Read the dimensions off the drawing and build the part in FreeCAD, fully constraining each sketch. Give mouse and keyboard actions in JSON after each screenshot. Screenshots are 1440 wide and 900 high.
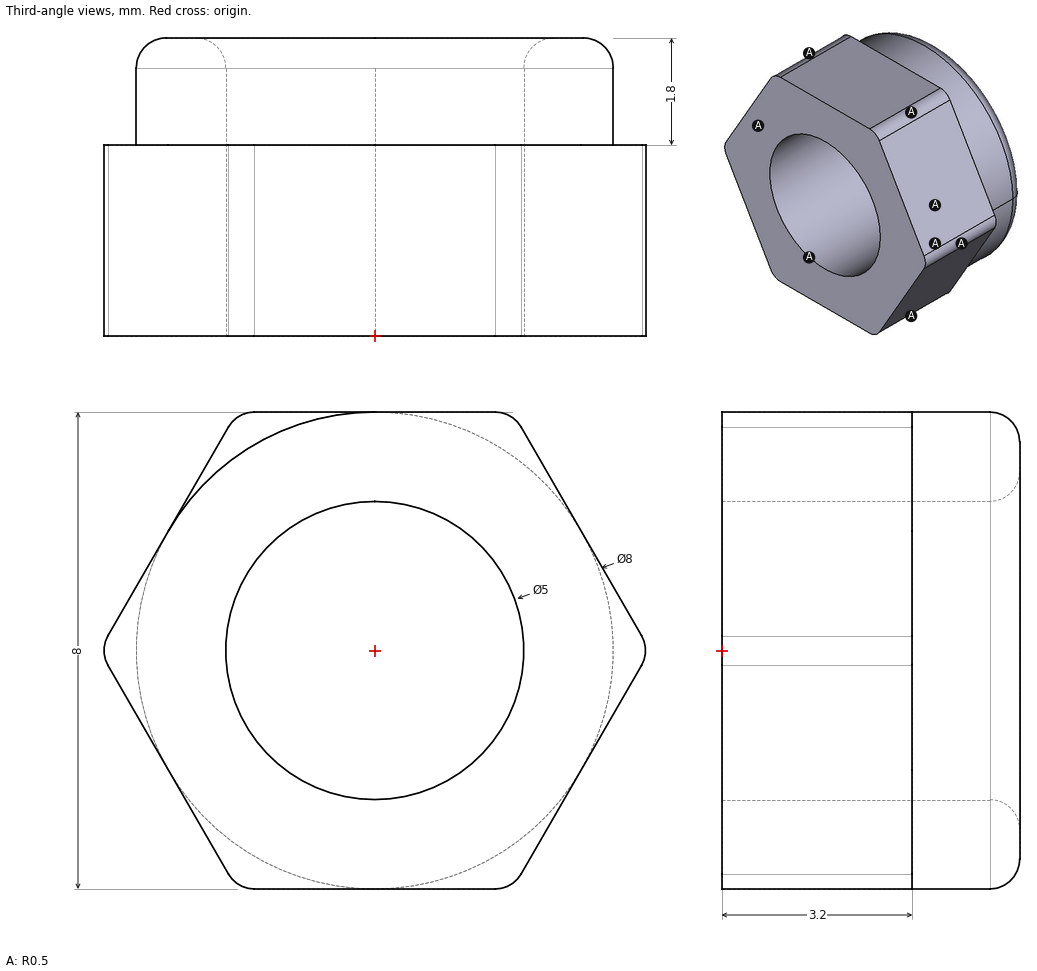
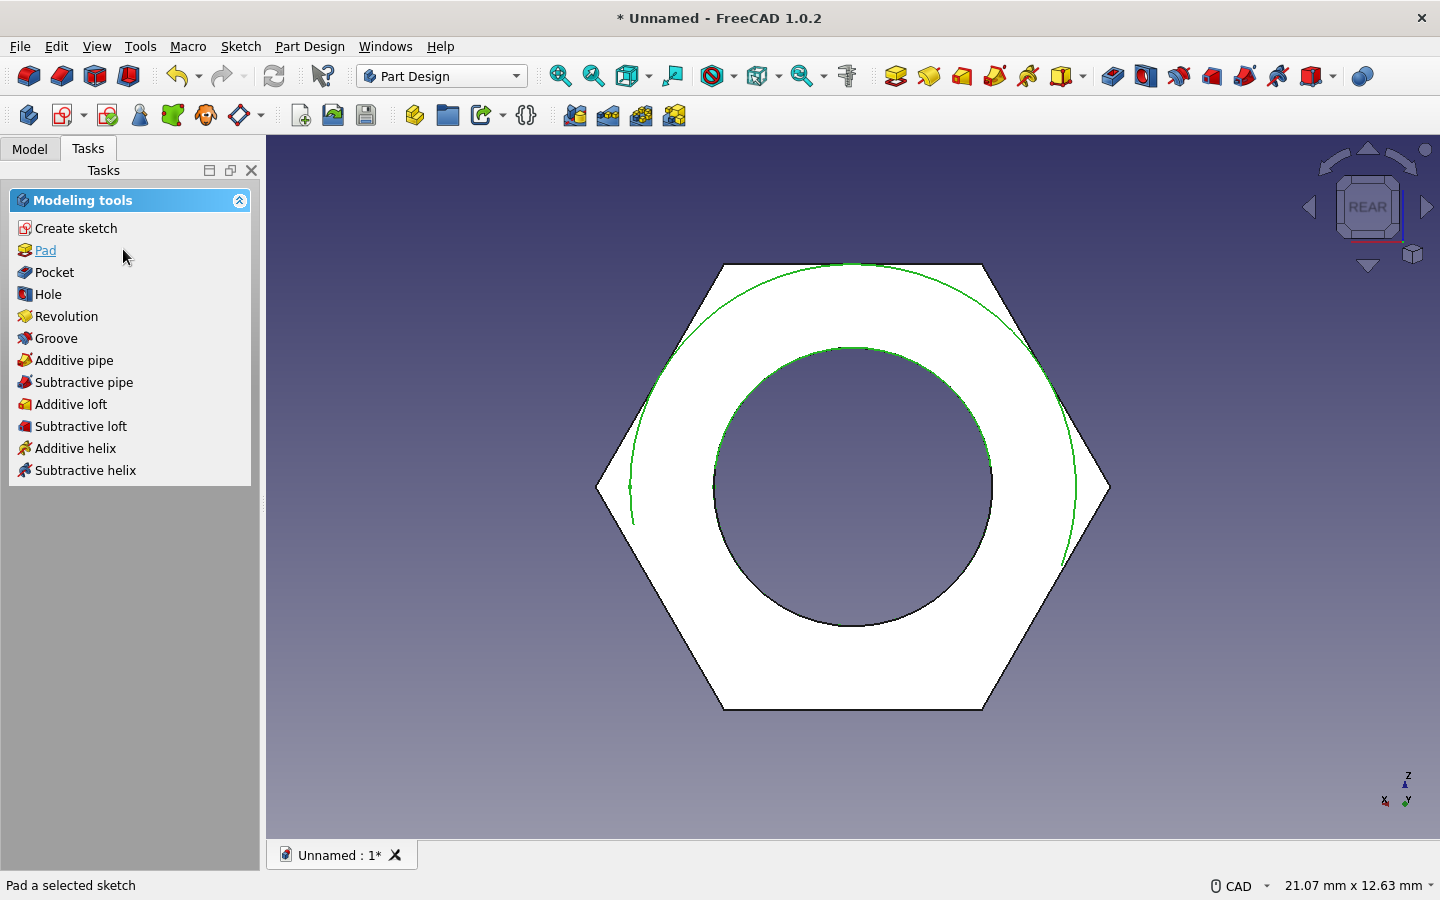
{"action": "left_click", "coordinate": [896, 76]}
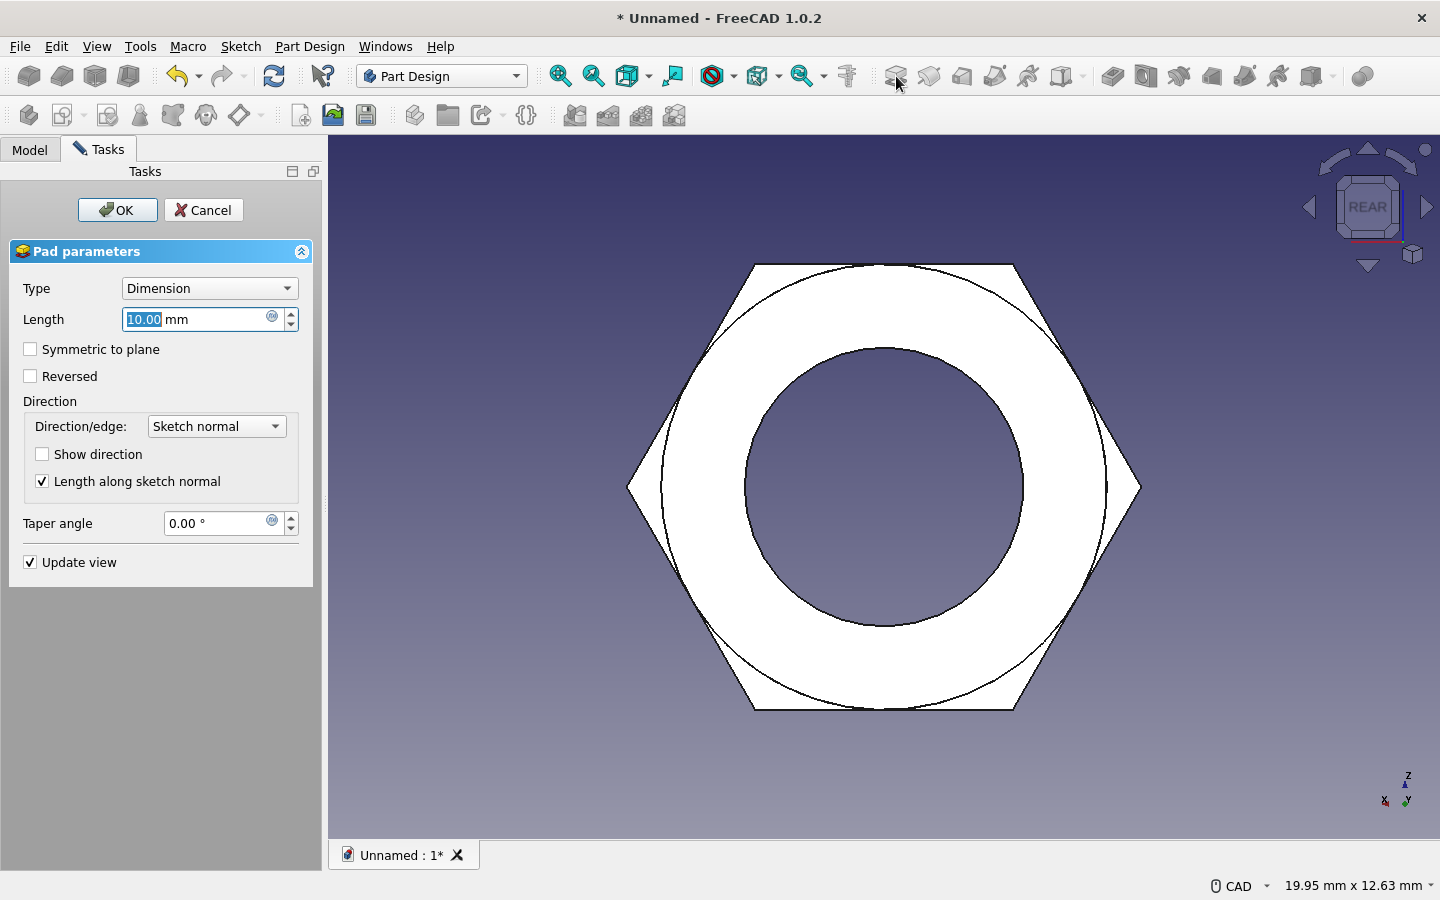
{"action": "type", "text": "1.8"}
{"action": "key", "text": "Tab"}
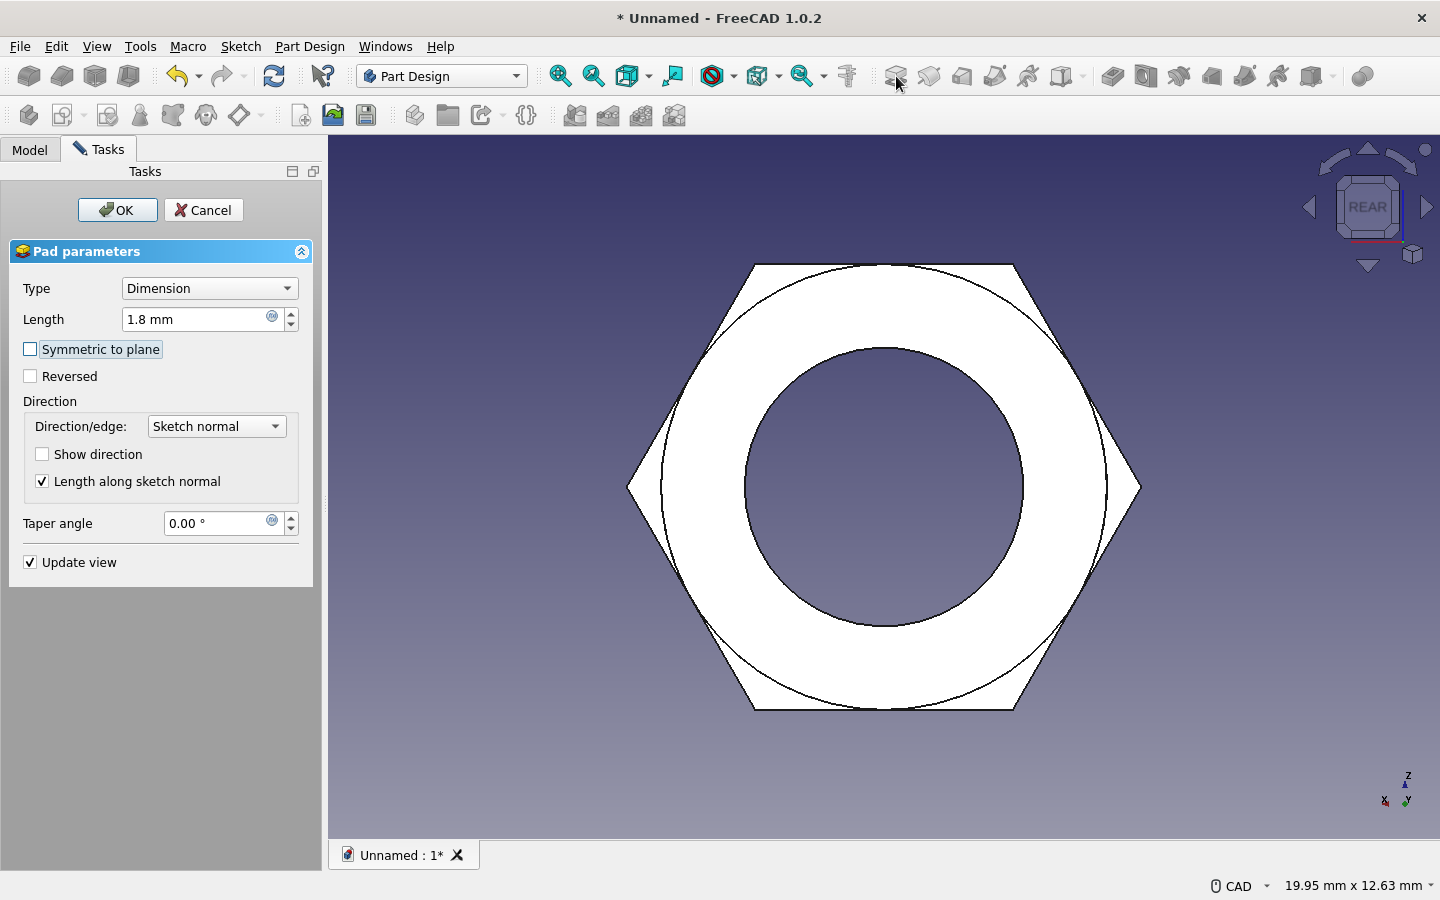
{"action": "left_click", "coordinate": [118, 210]}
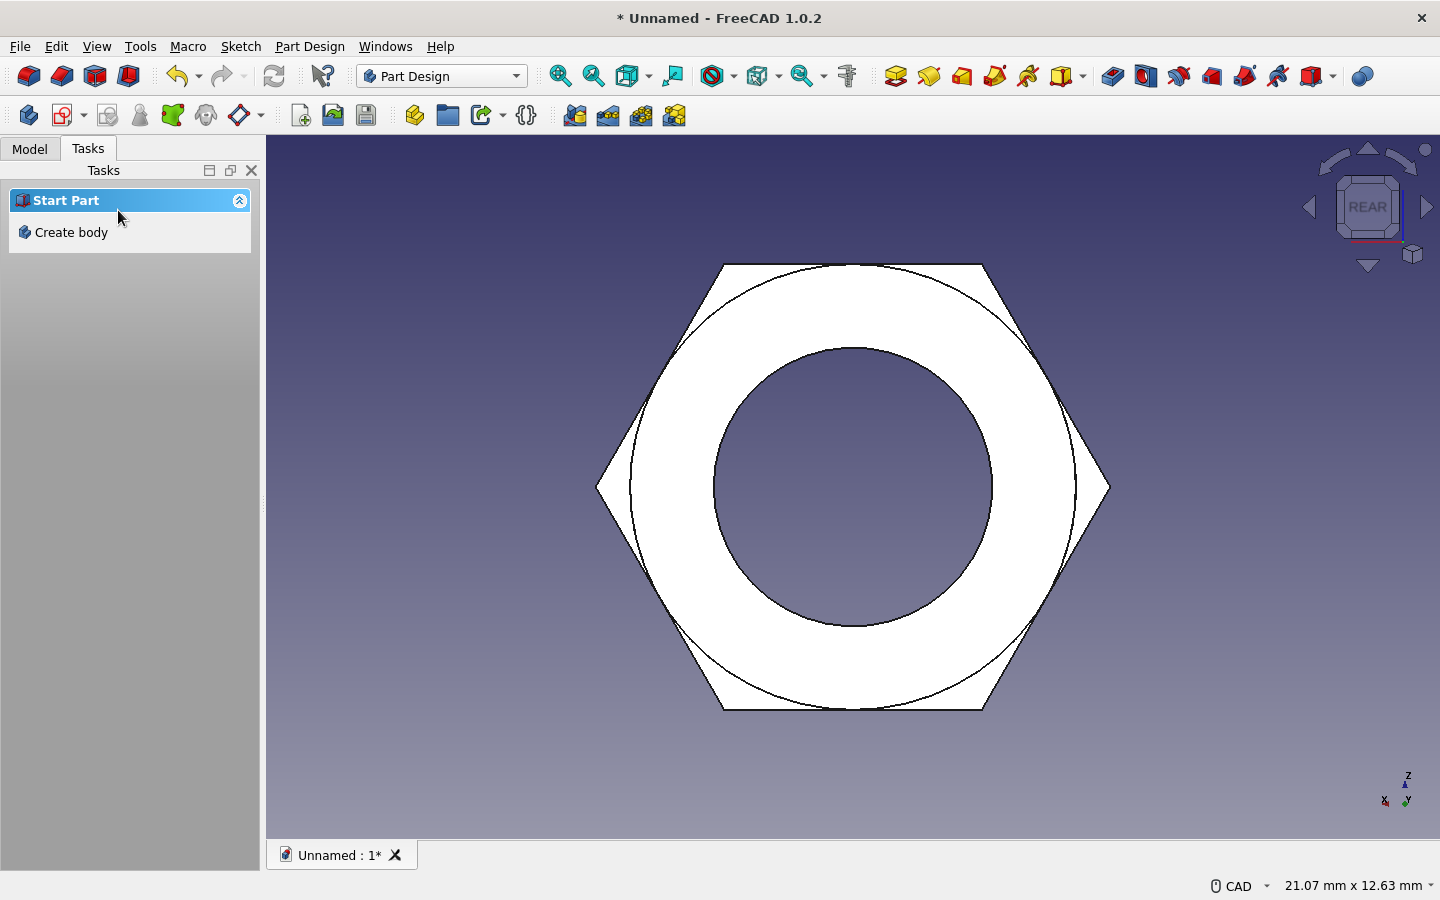
{"action": "left_click", "coordinate": [1076, 486]}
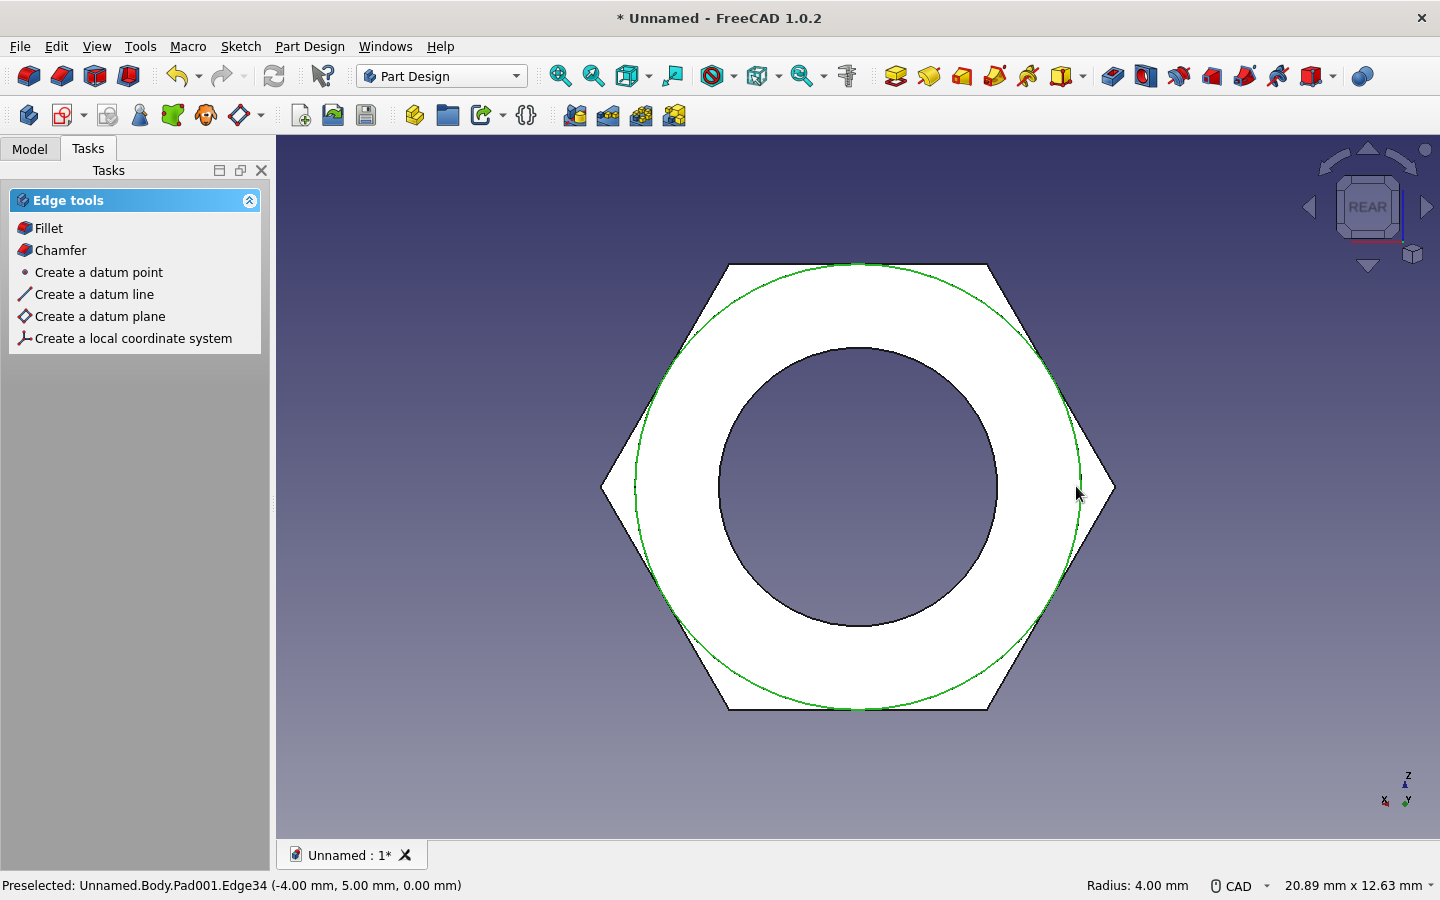
{"action": "left_click", "coordinate": [971, 404], "text": "ctrl"}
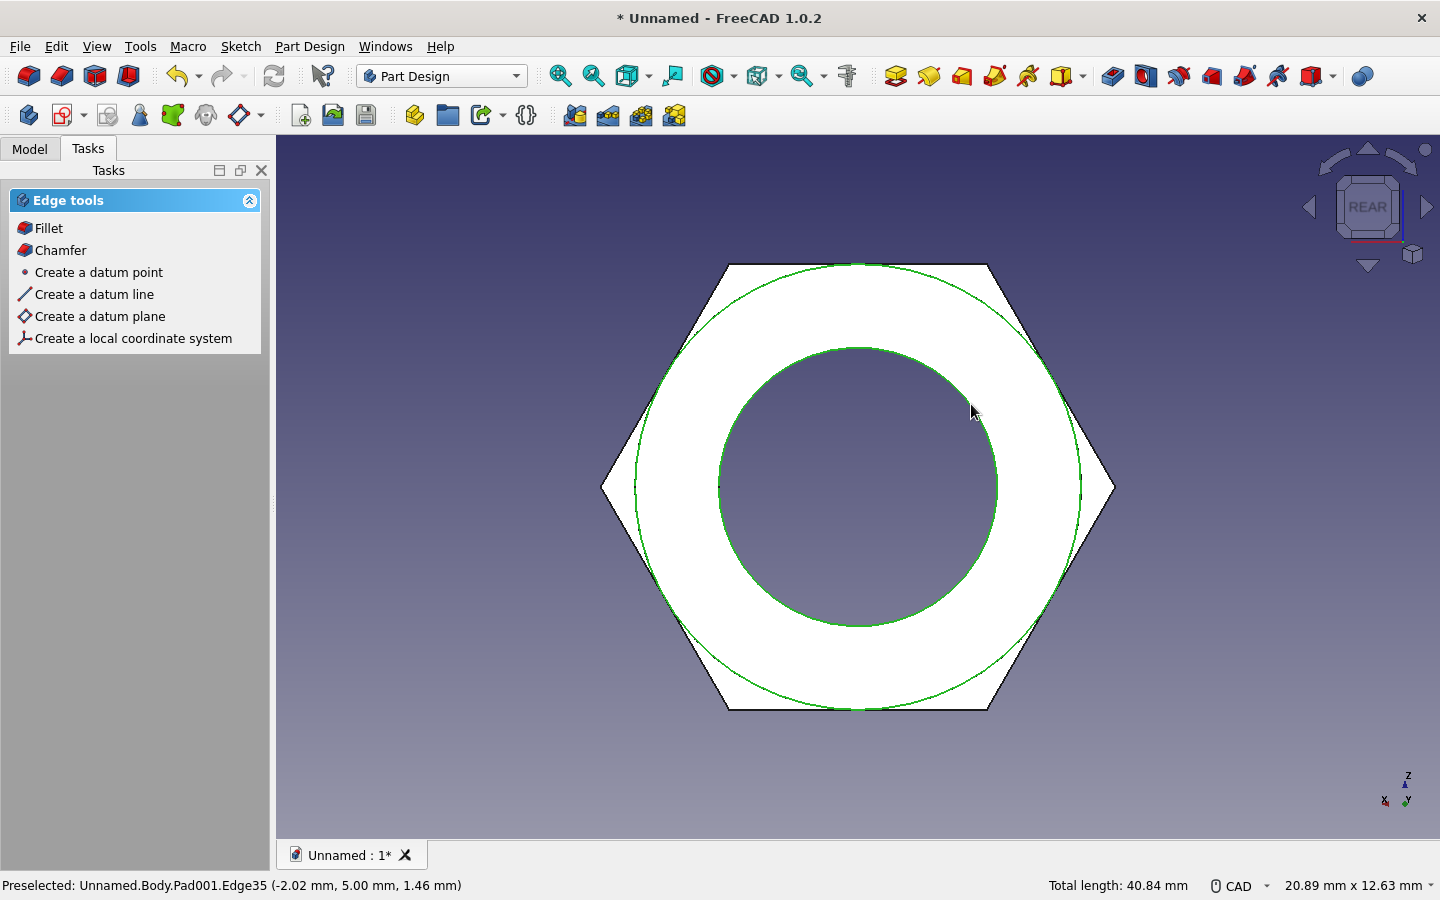
{"action": "key", "text": "0"}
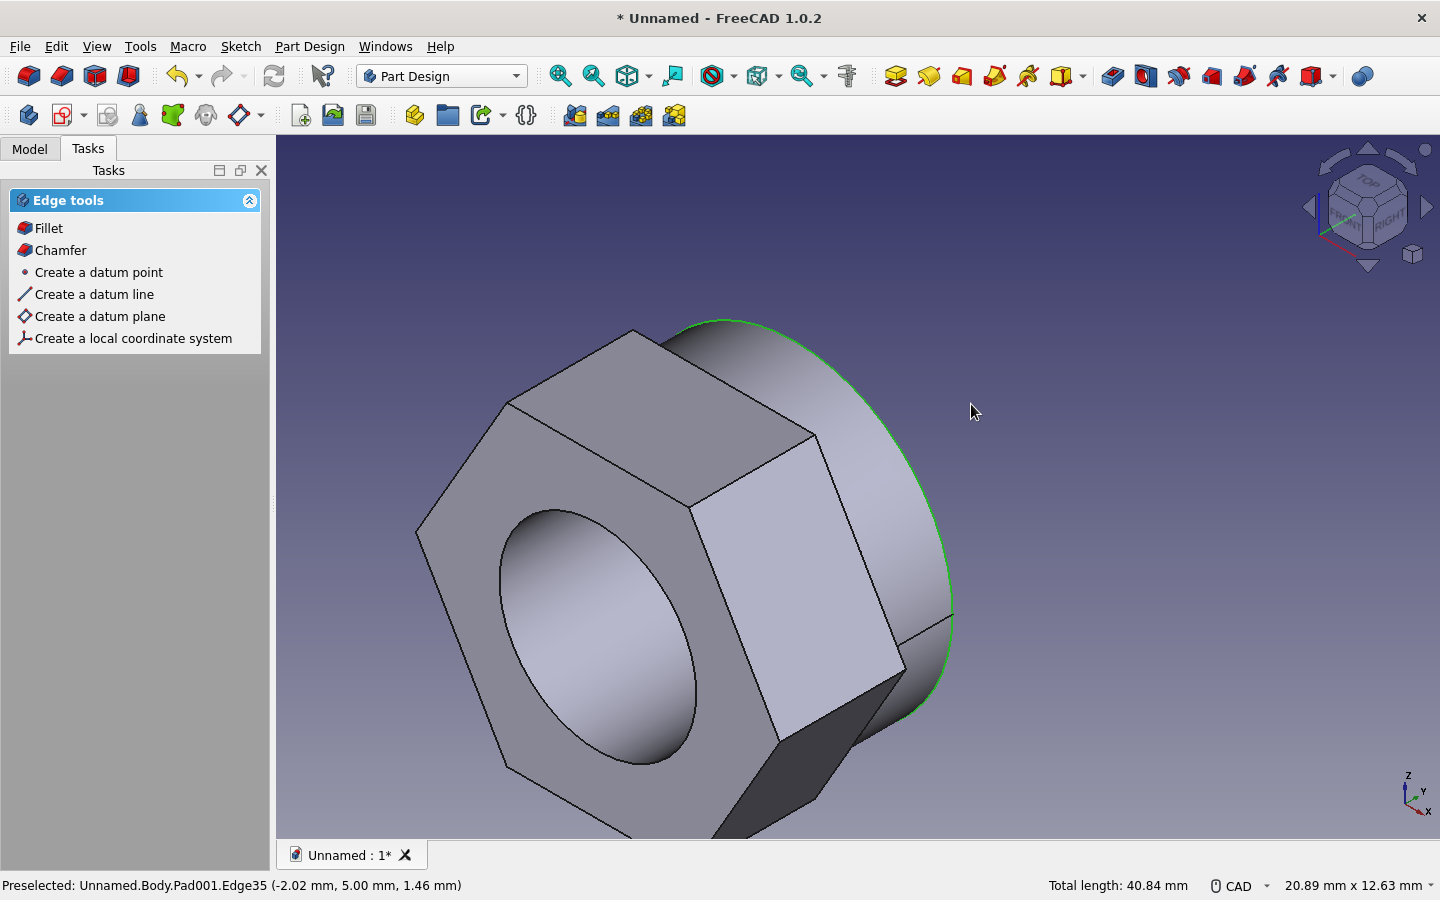
{"action": "left_click", "coordinate": [561, 76]}